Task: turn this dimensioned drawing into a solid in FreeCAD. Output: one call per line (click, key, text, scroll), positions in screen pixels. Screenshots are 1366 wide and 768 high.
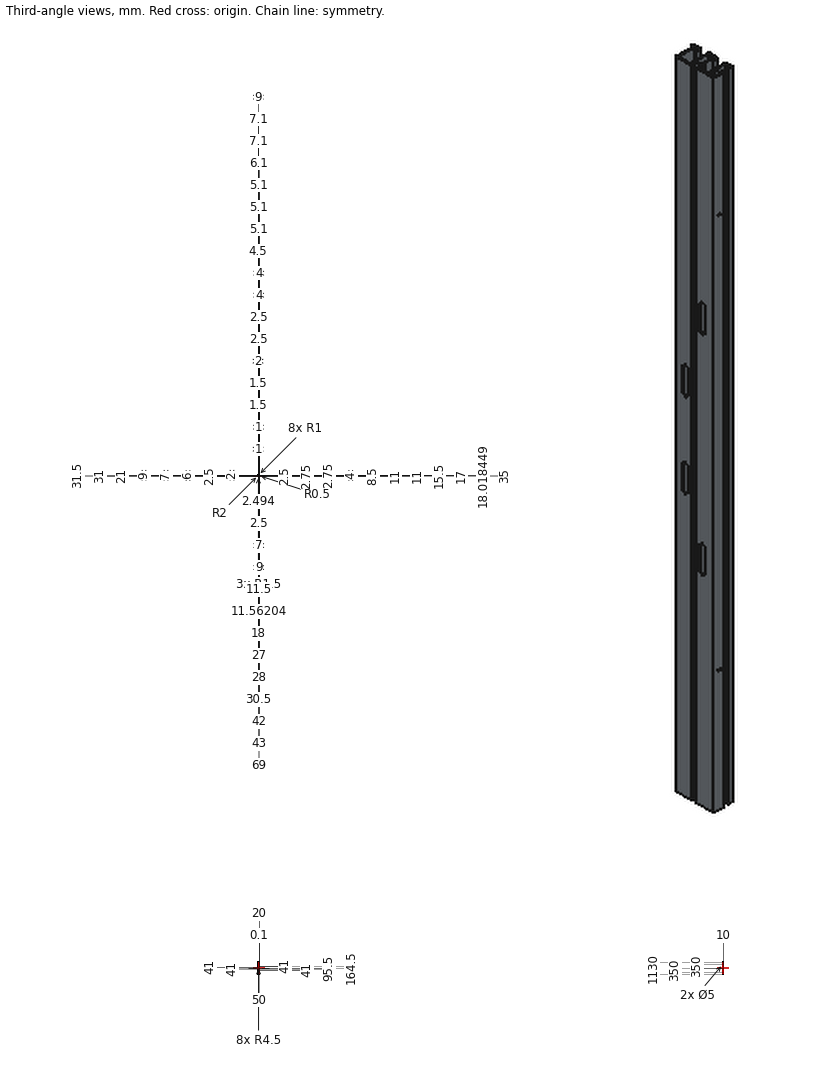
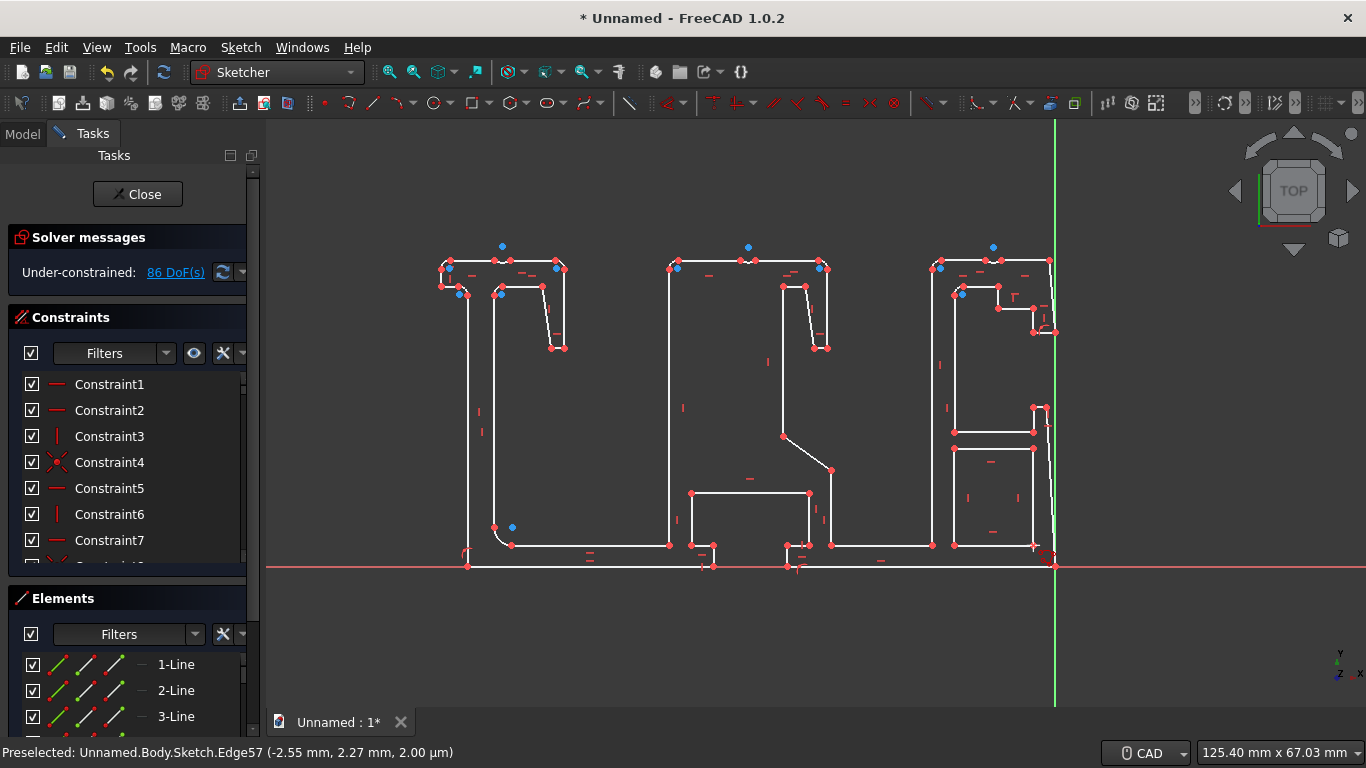
click(788, 470)
click(687, 470)
click(687, 286)
click(766, 286)
click(766, 444)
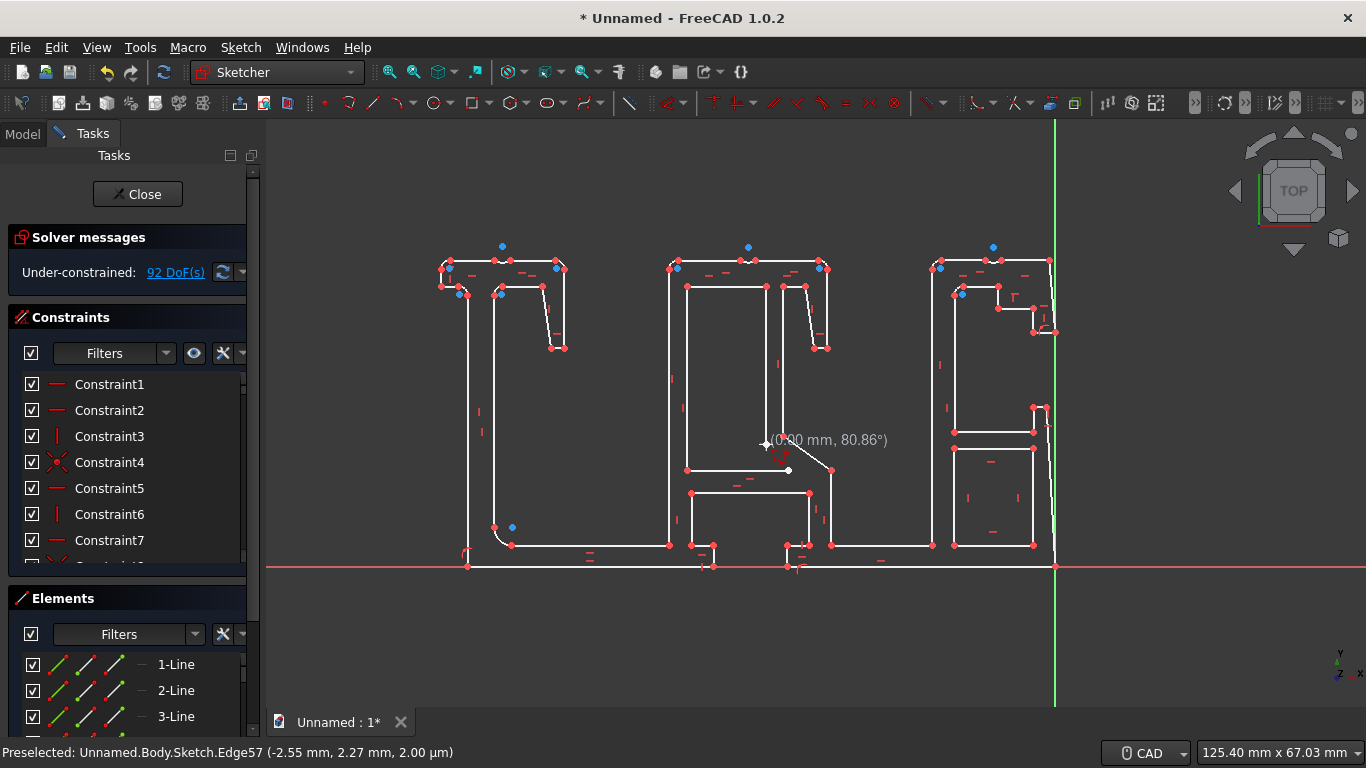
scroll(791, 462, up, 4)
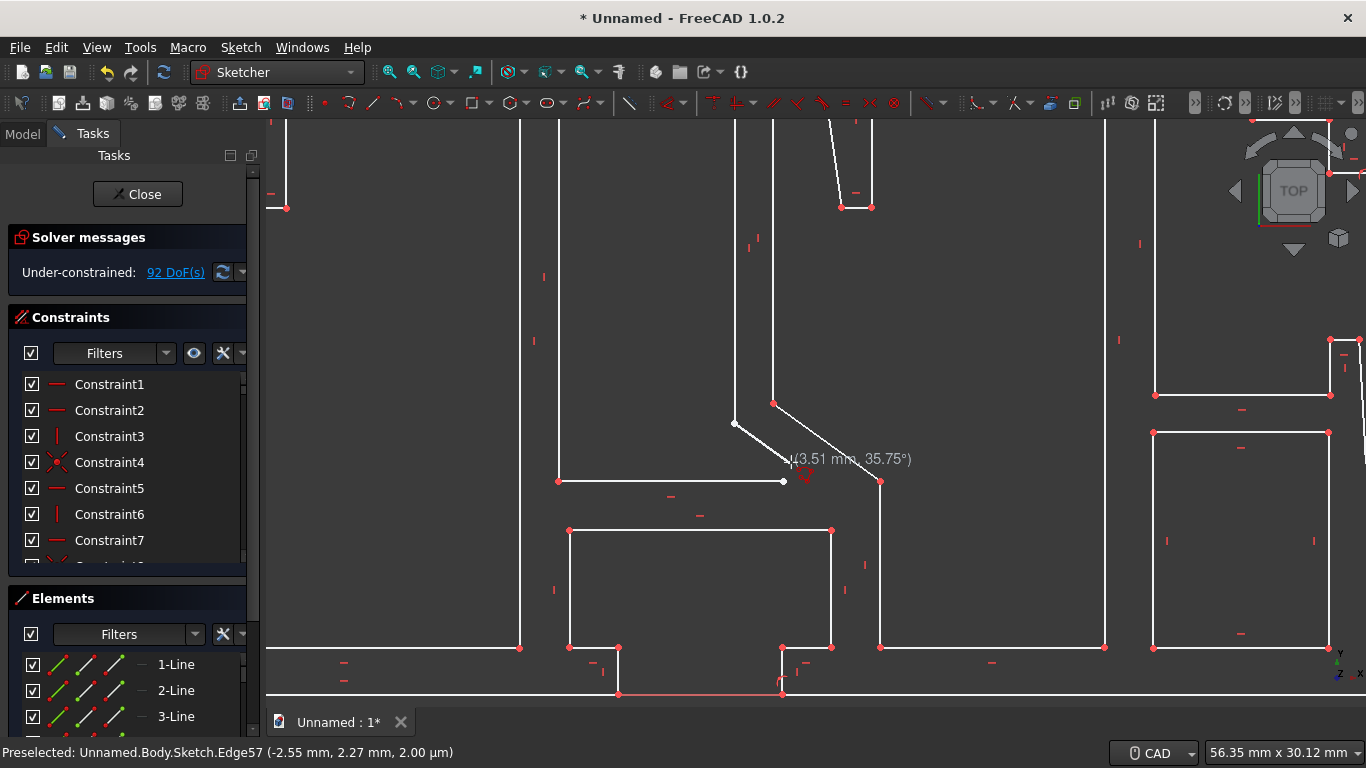
click(790, 462)
right_click(790, 462)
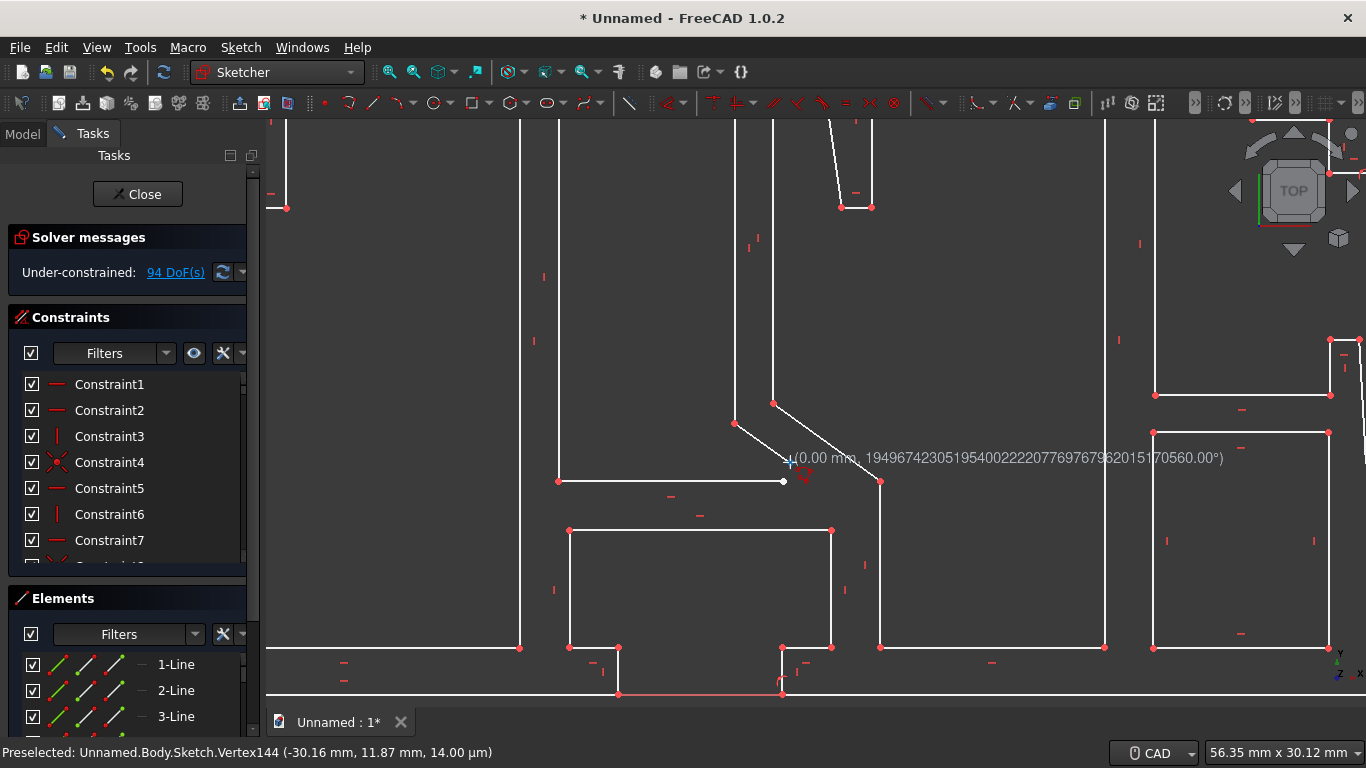
click(398, 104)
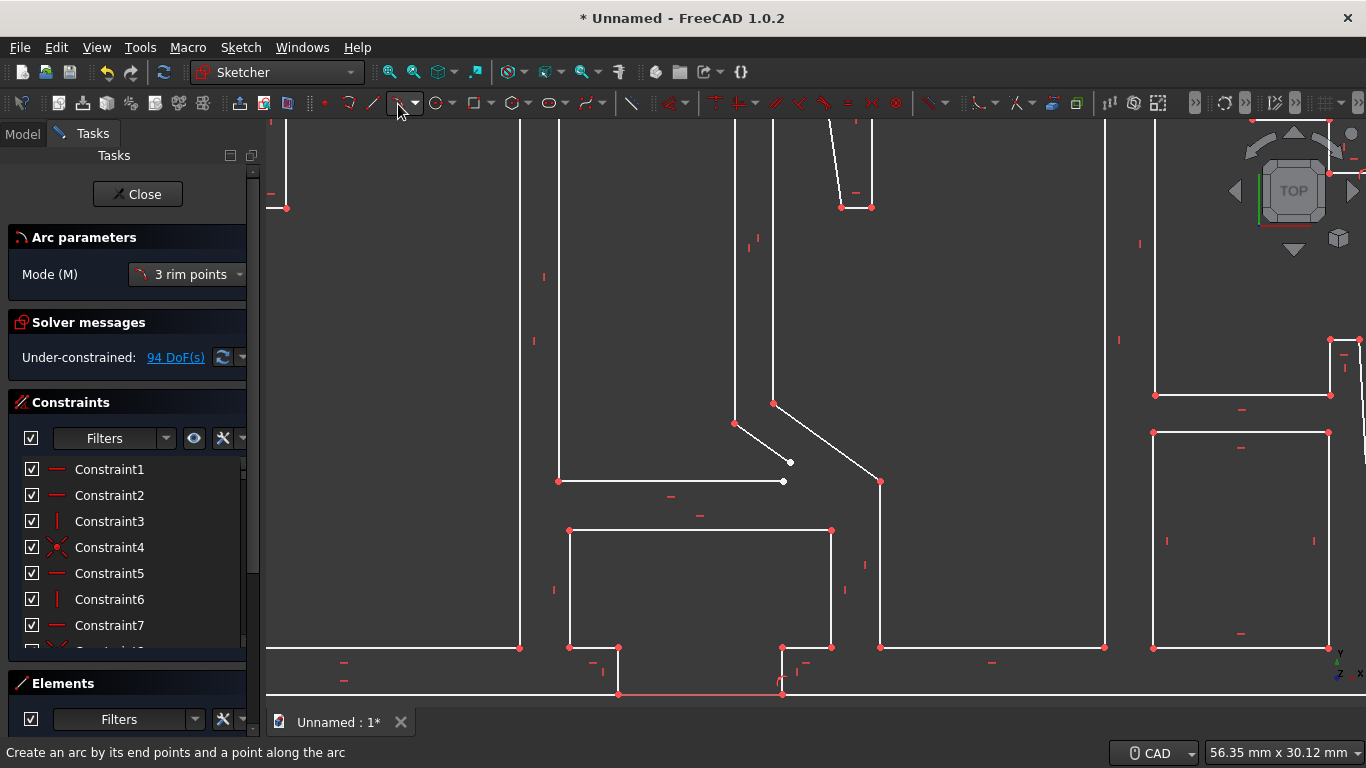
click(790, 463)
click(784, 481)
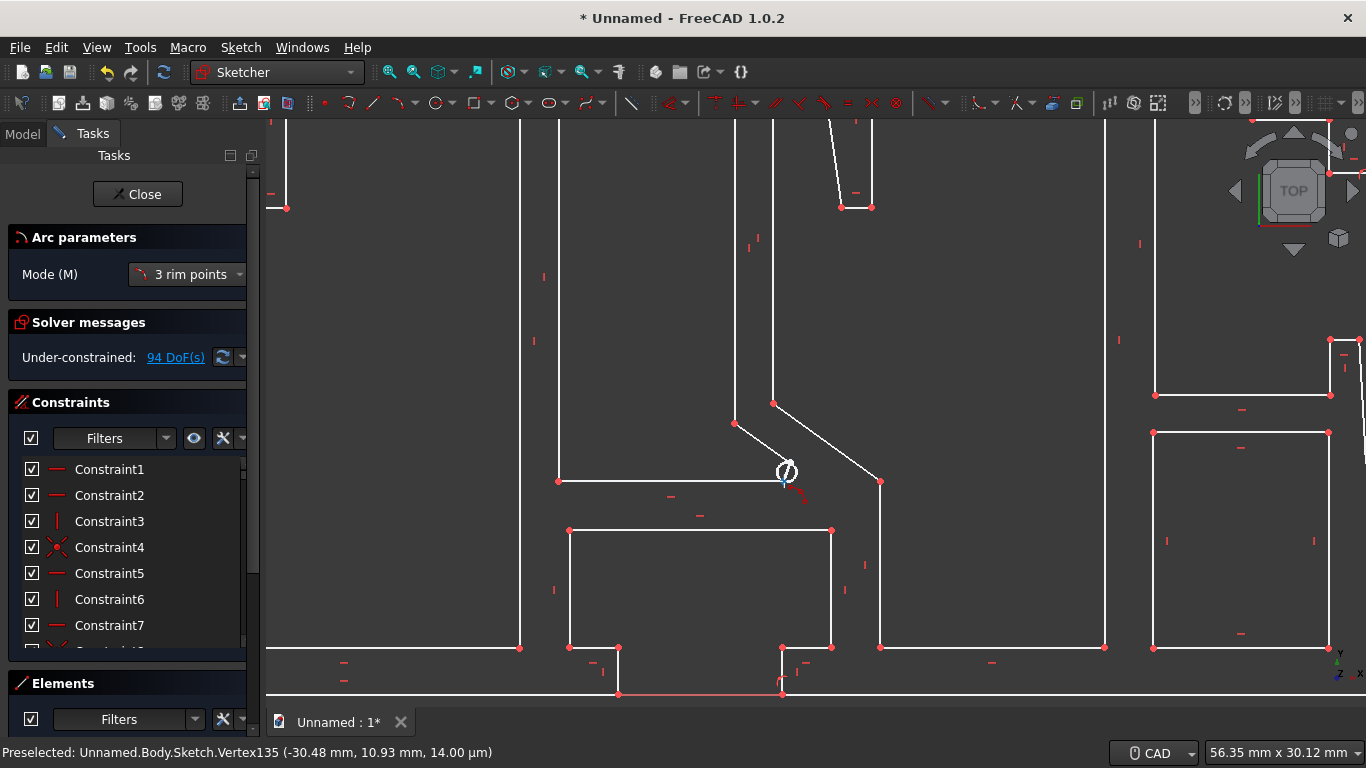
scroll(794, 473, up, 5)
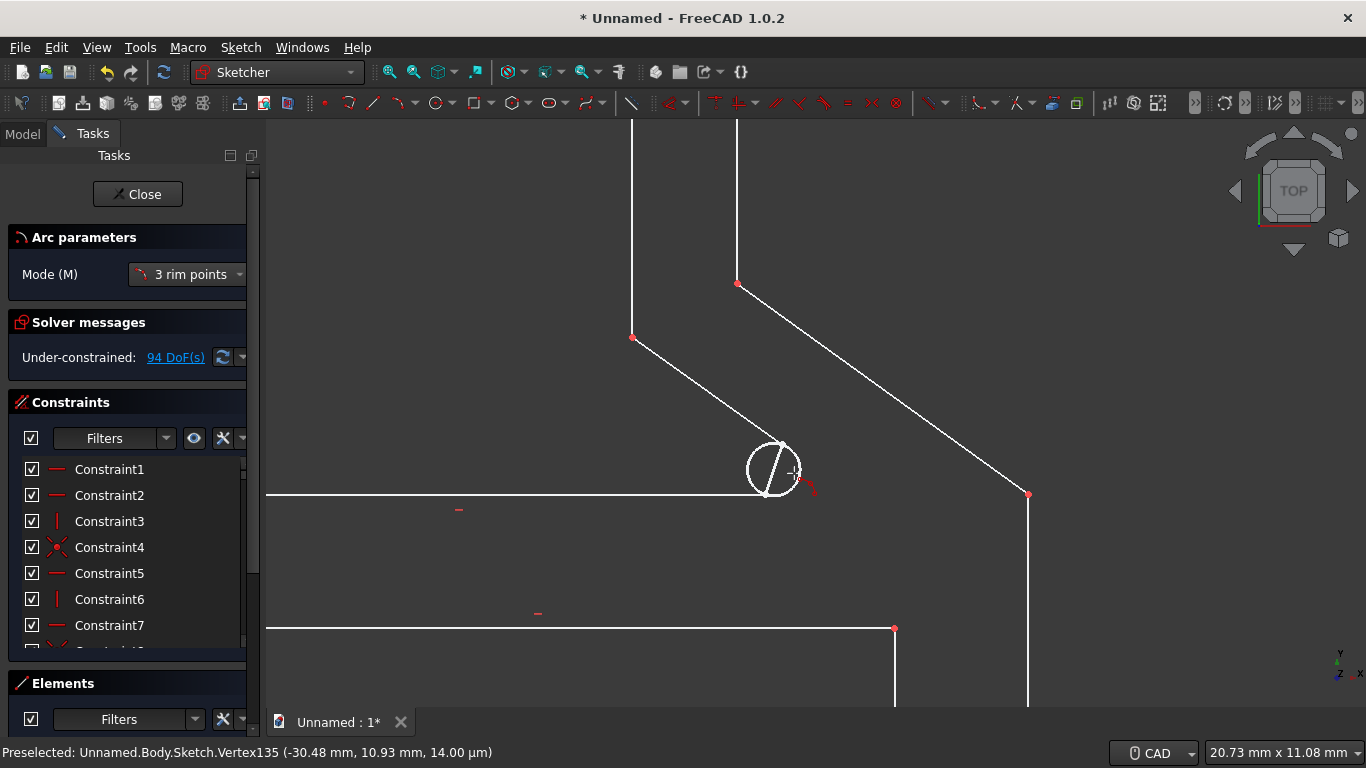
click(793, 473)
key(Escape)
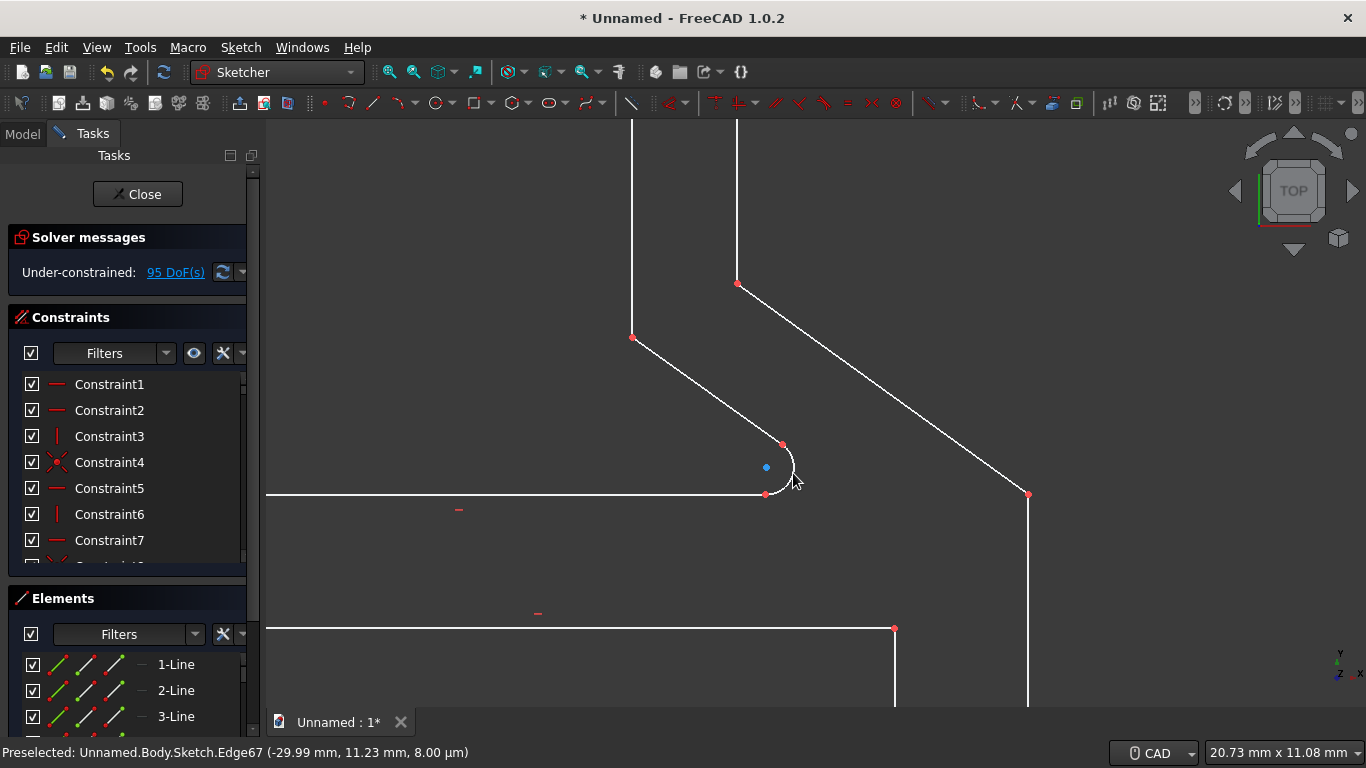
scroll(792, 466, down, 9)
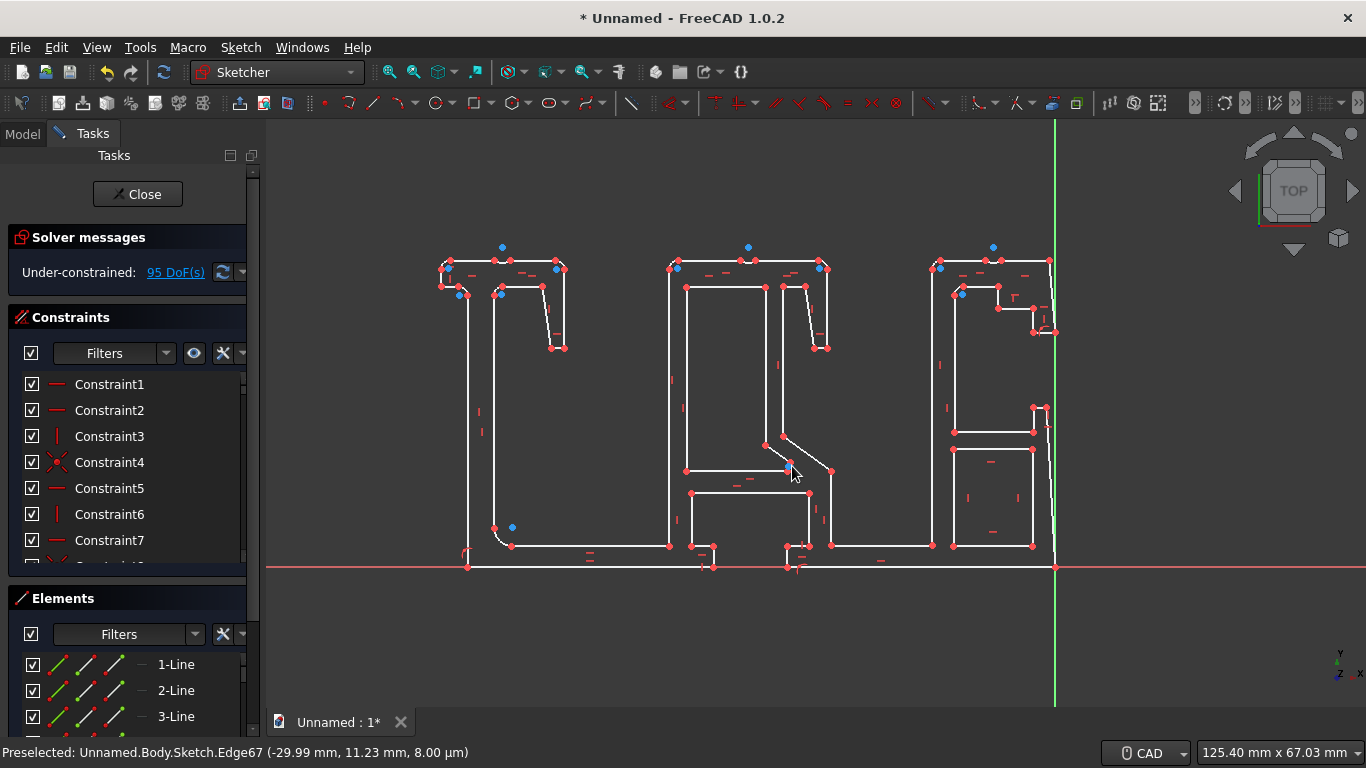
click(800, 261)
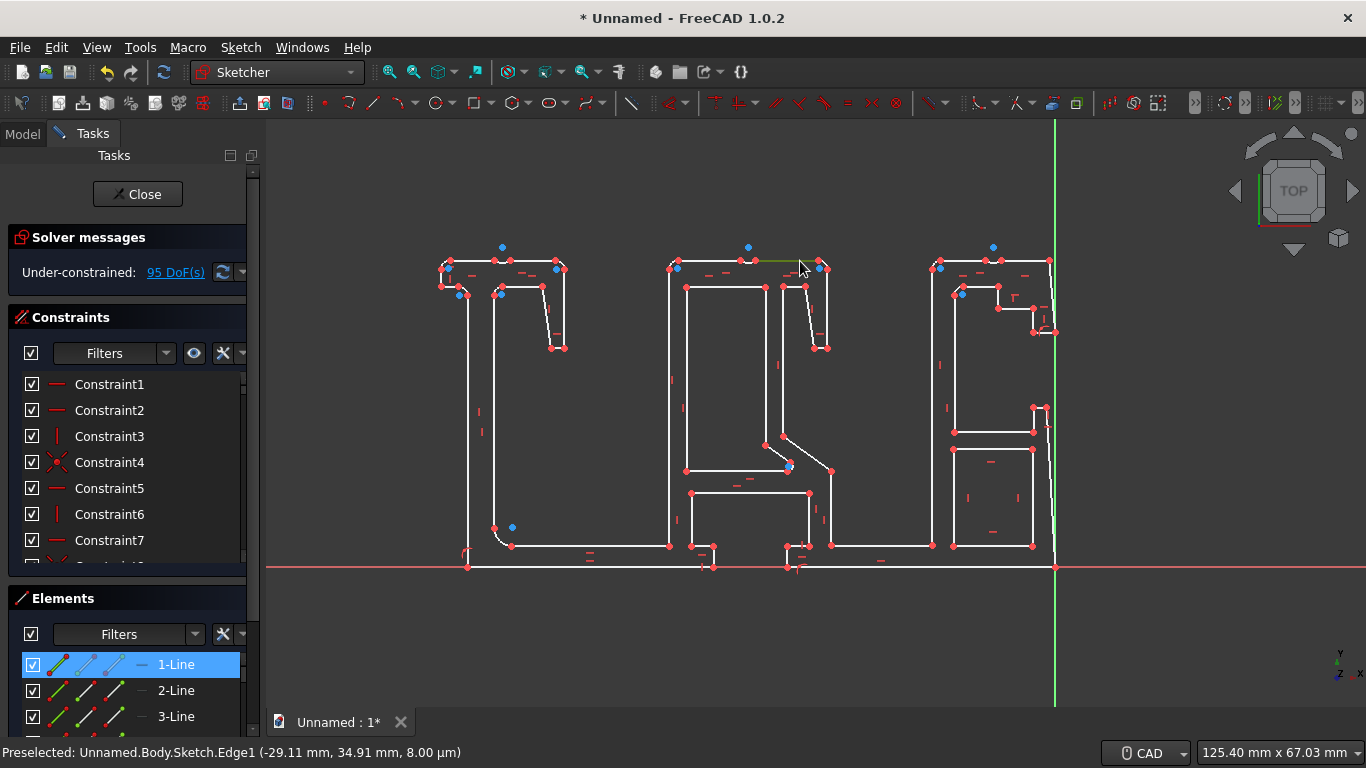
scroll(825, 263, up, 4)